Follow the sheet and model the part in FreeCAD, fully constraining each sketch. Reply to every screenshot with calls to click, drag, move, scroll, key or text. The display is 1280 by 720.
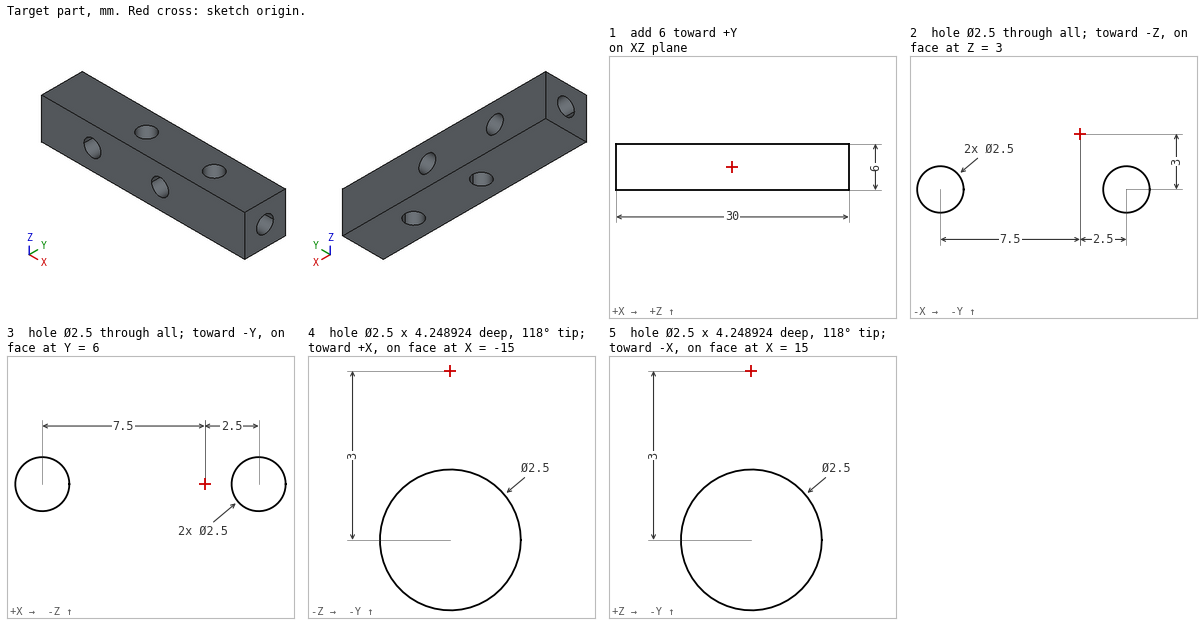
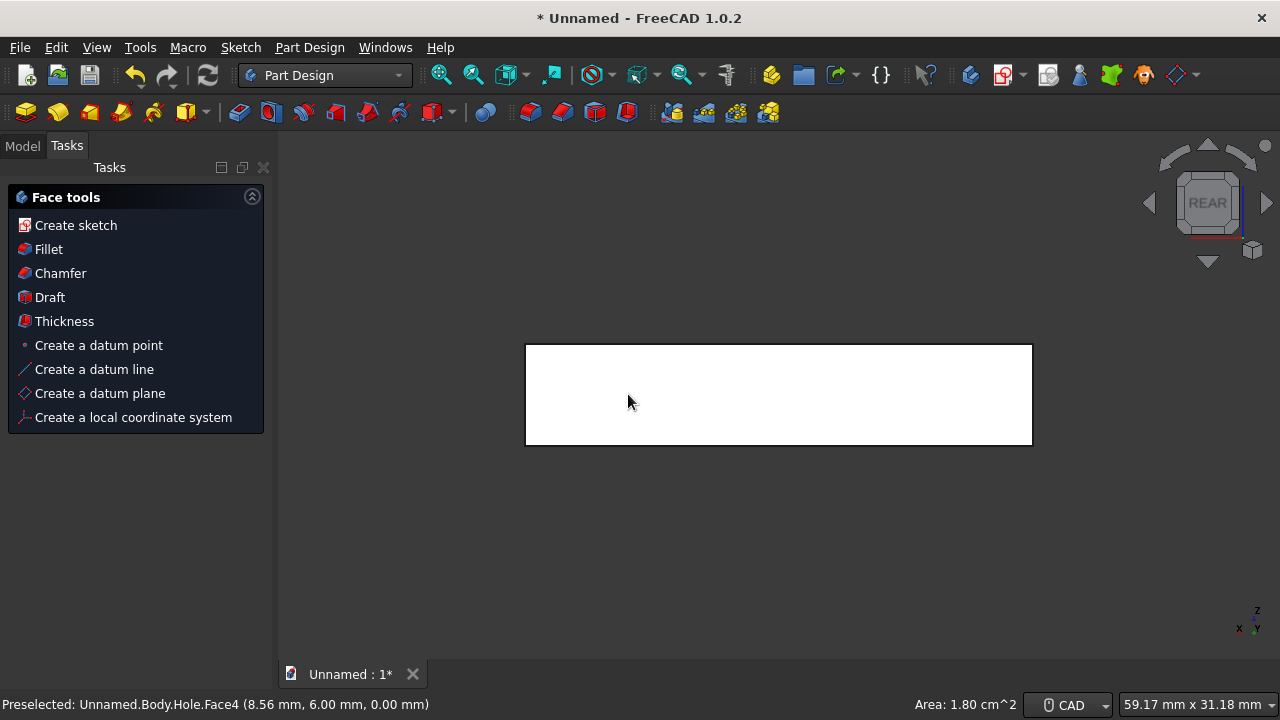
click(1004, 76)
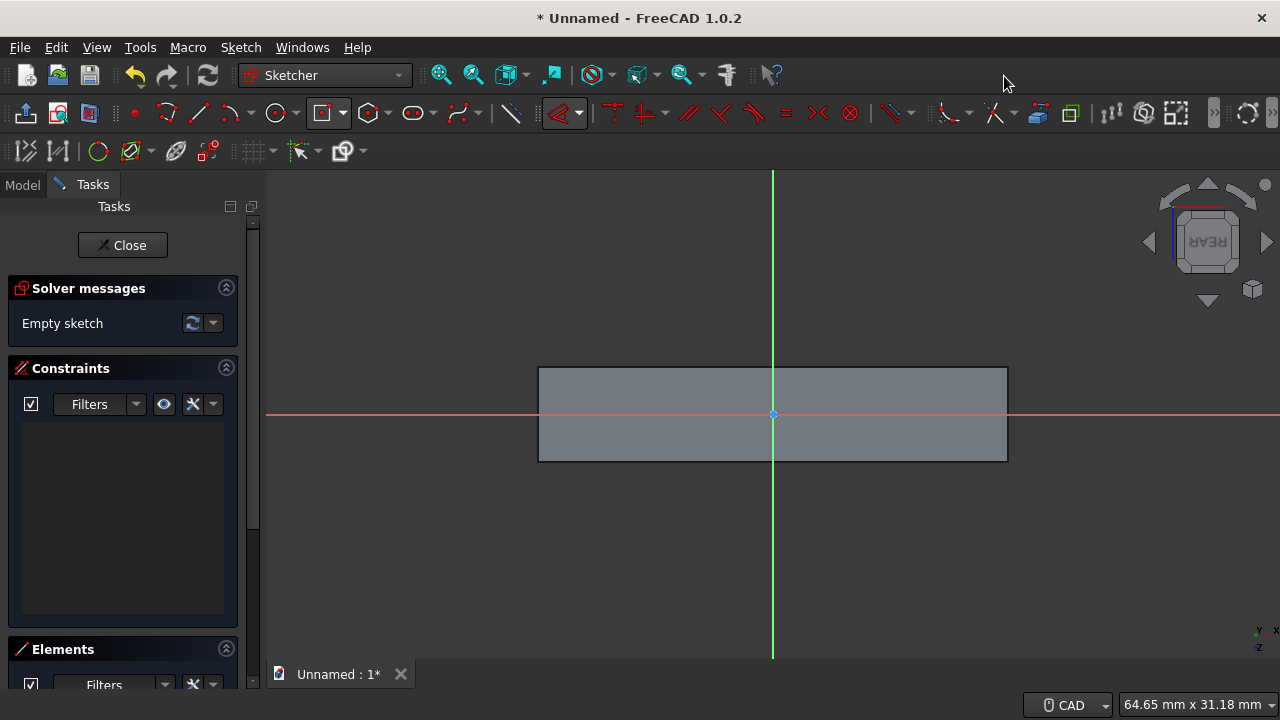
scroll(751, 414, up, 5)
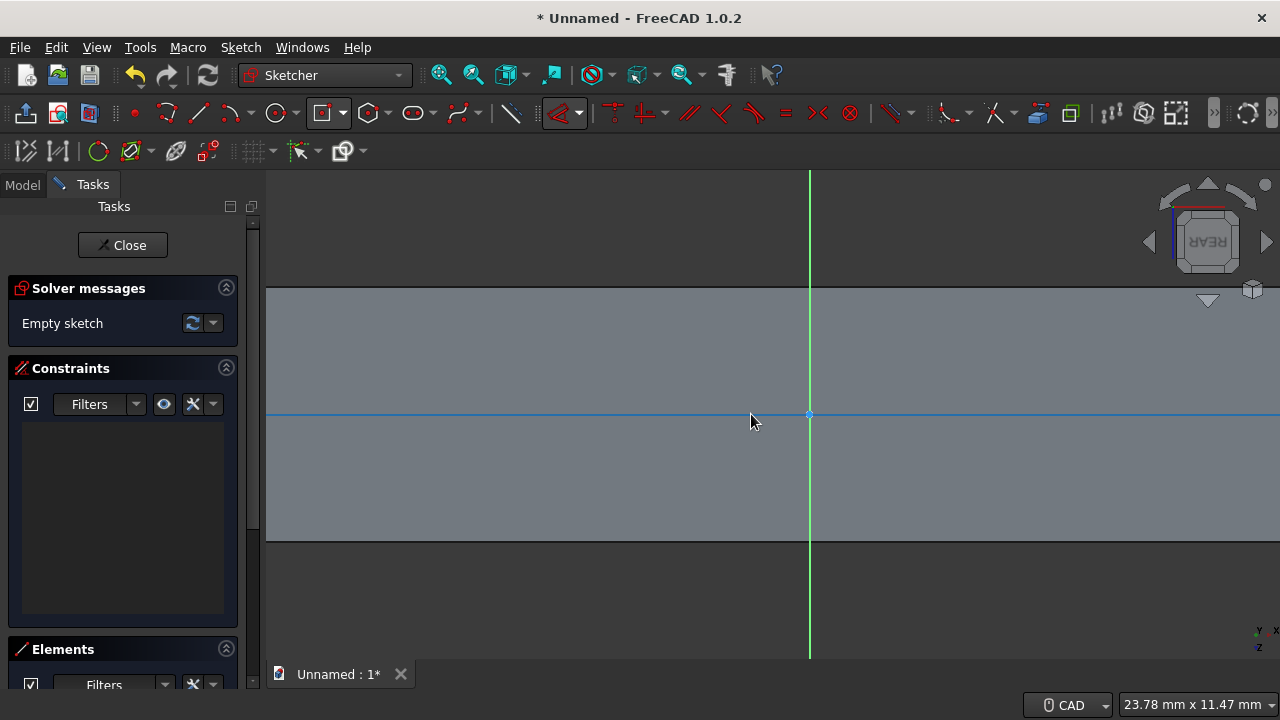
click(276, 114)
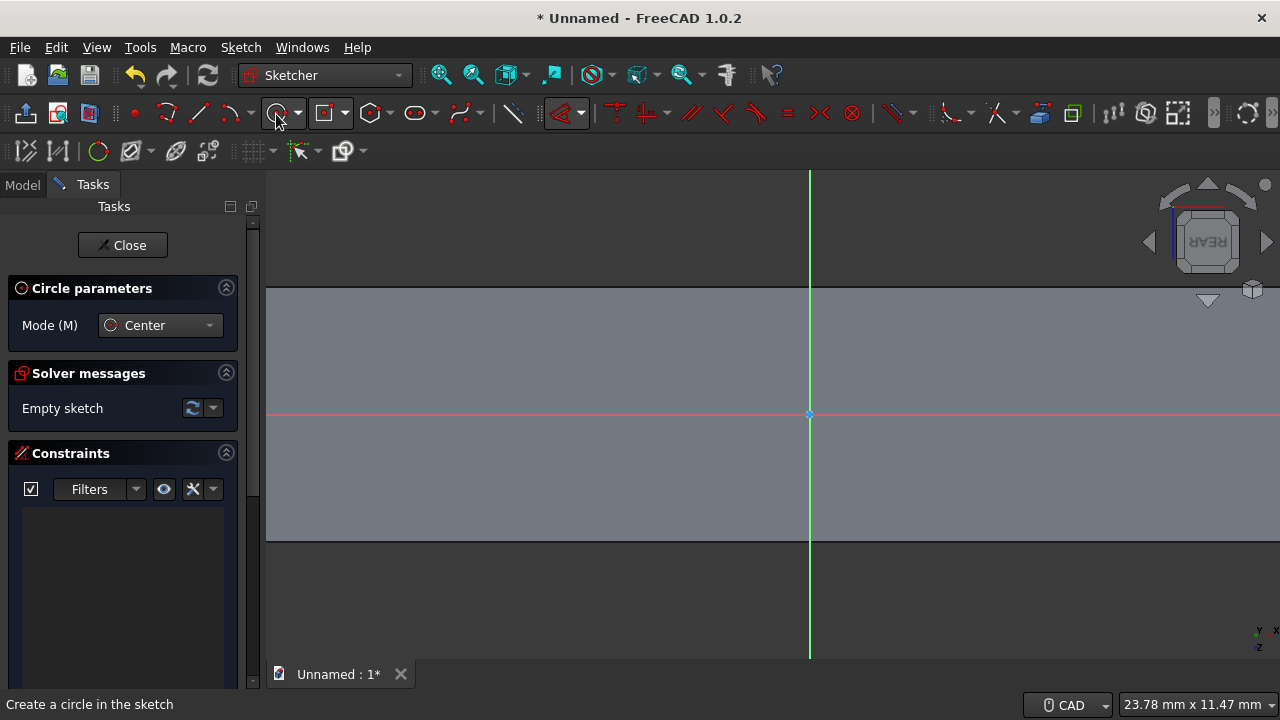
click(917, 414)
move(954, 377)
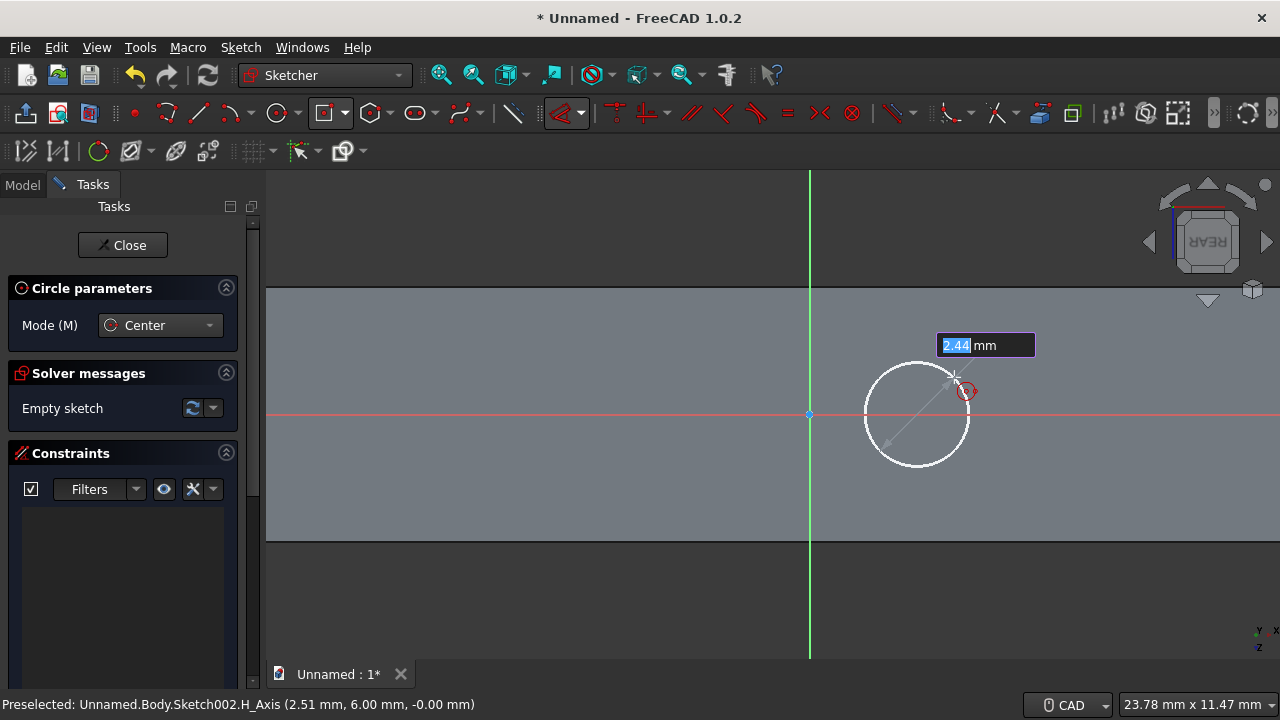
text(2.5)
key(Return)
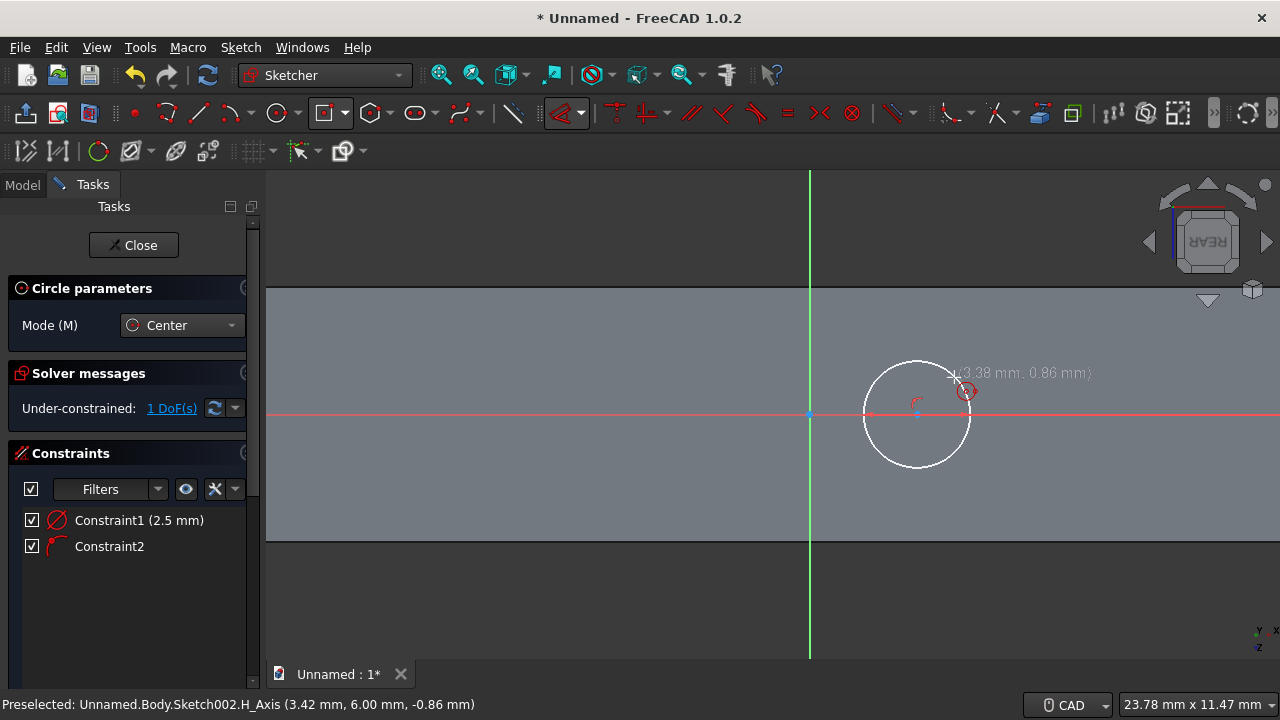
click(490, 414)
move(528, 377)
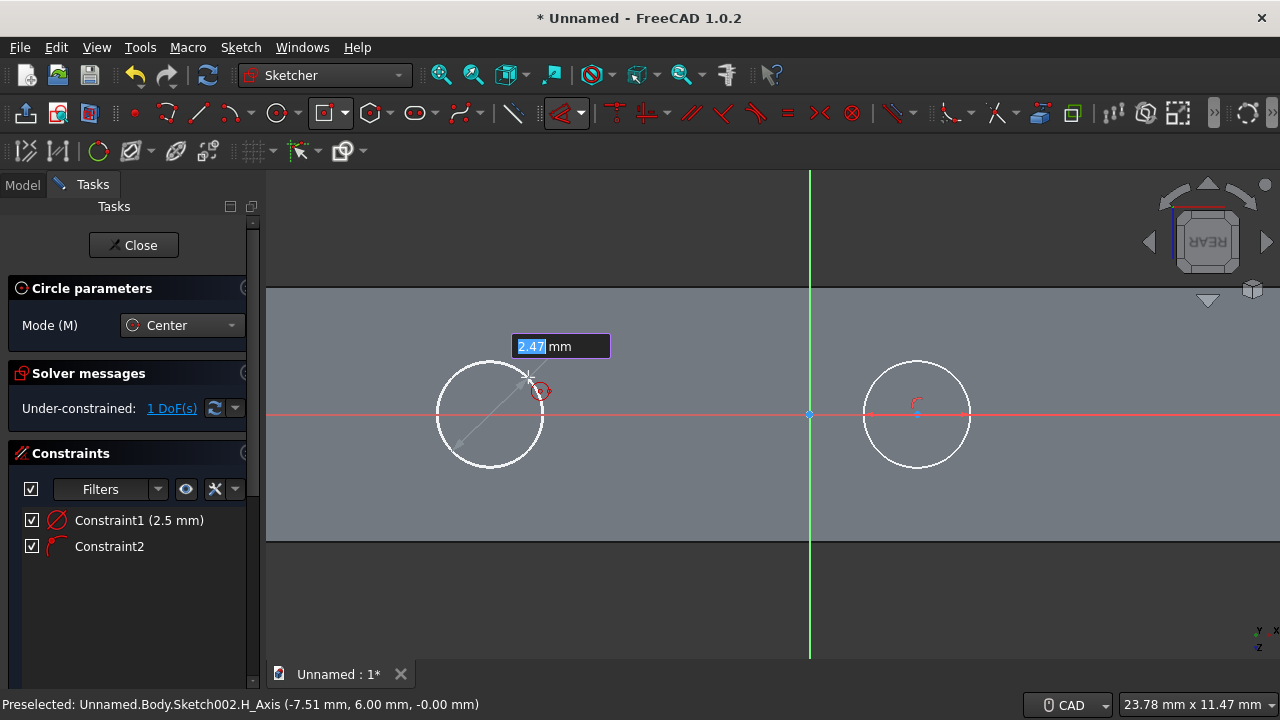
text(2.5)
key(Return)
key(Escape)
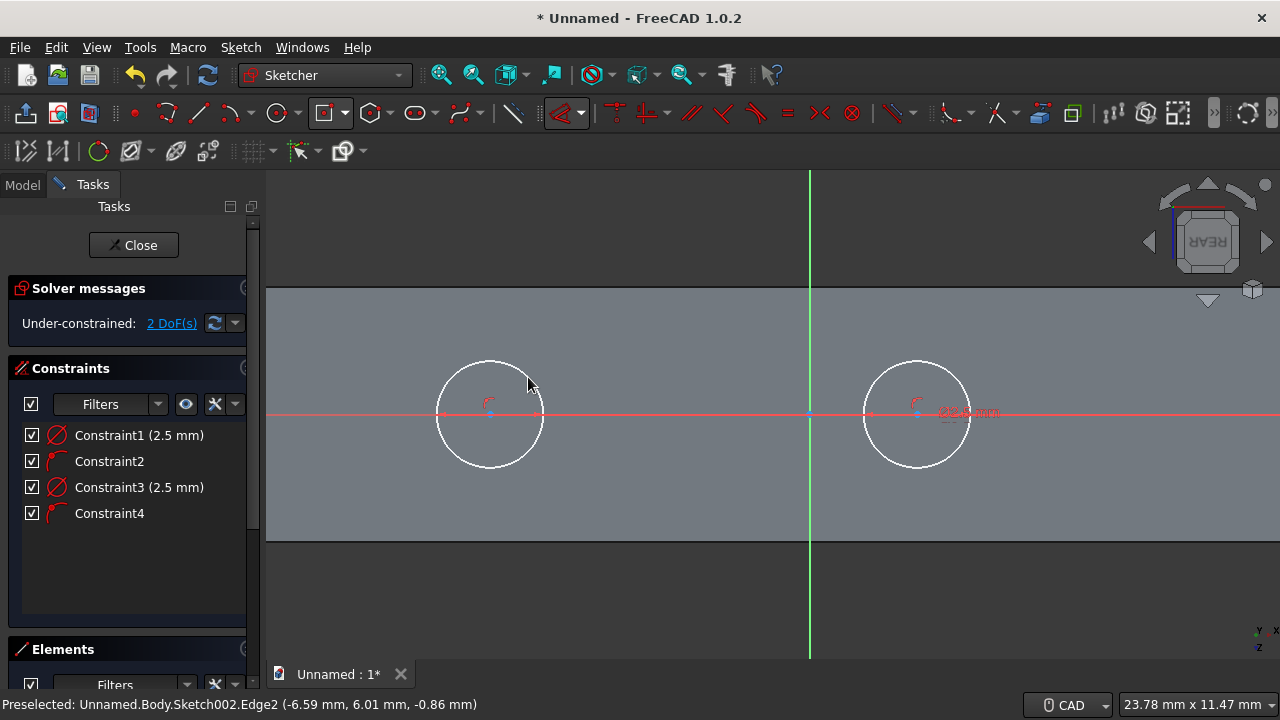
click(917, 414)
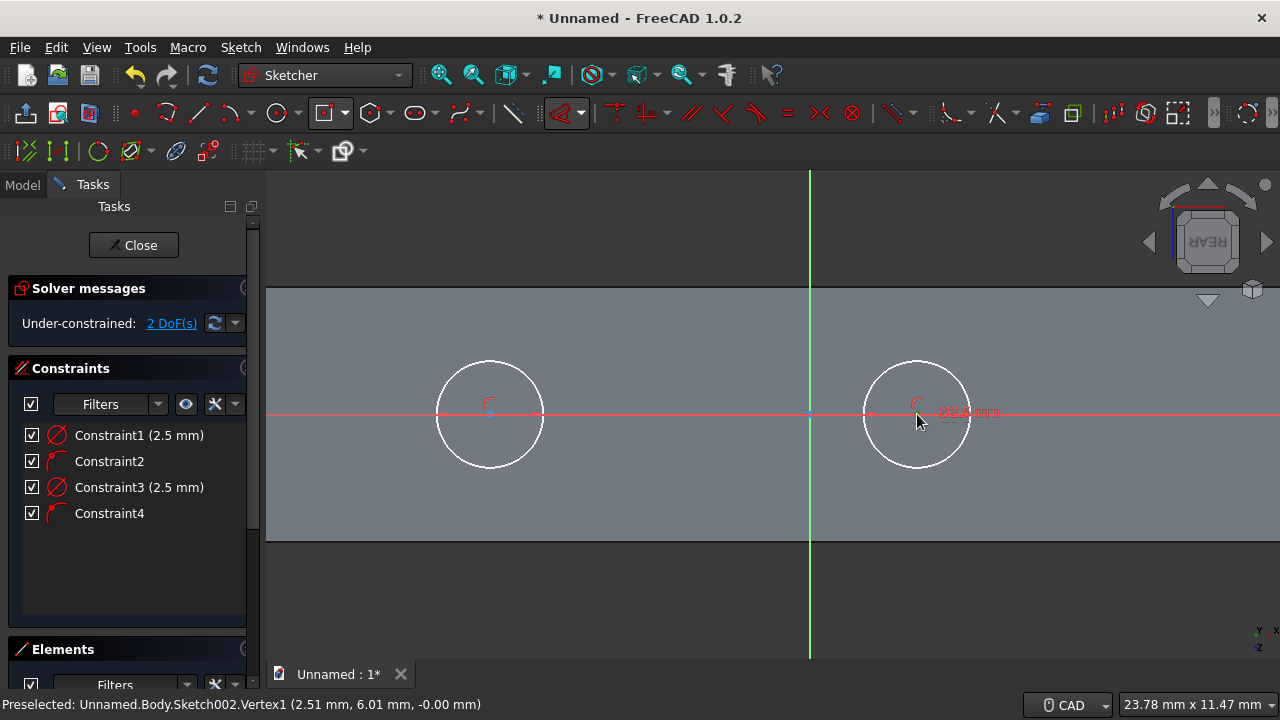
key(l)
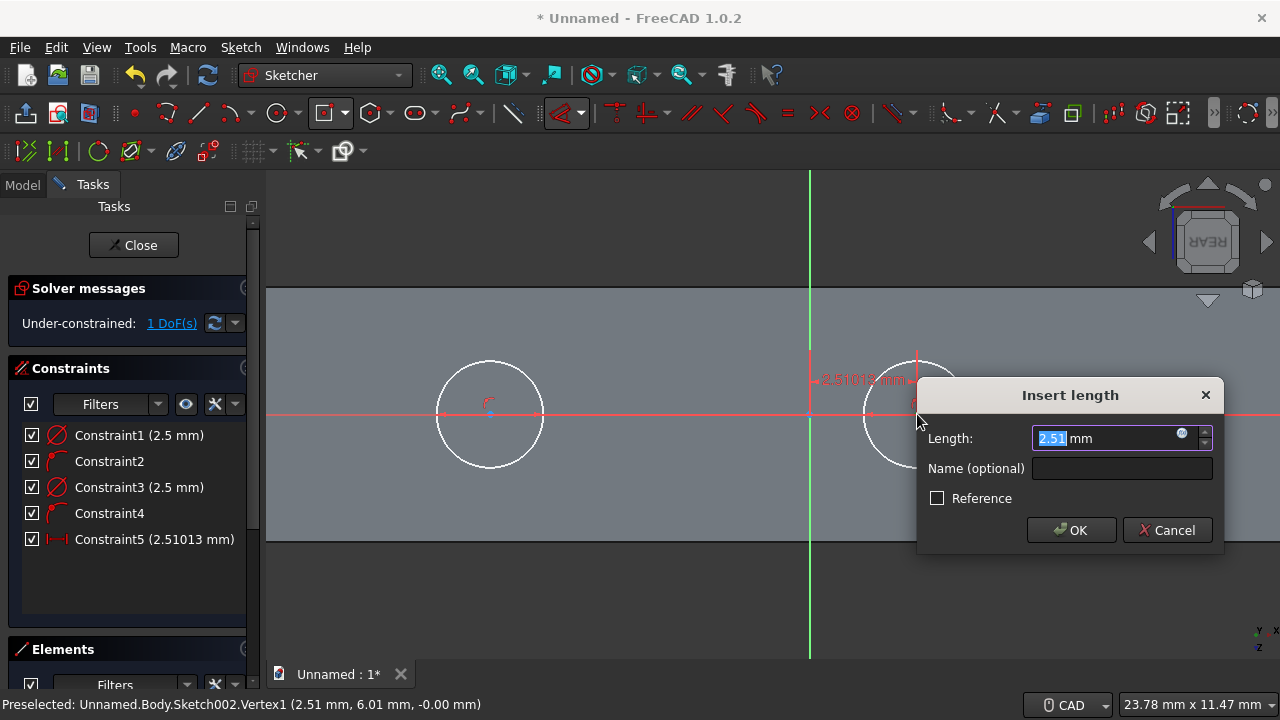
text(2.5)
key(Return)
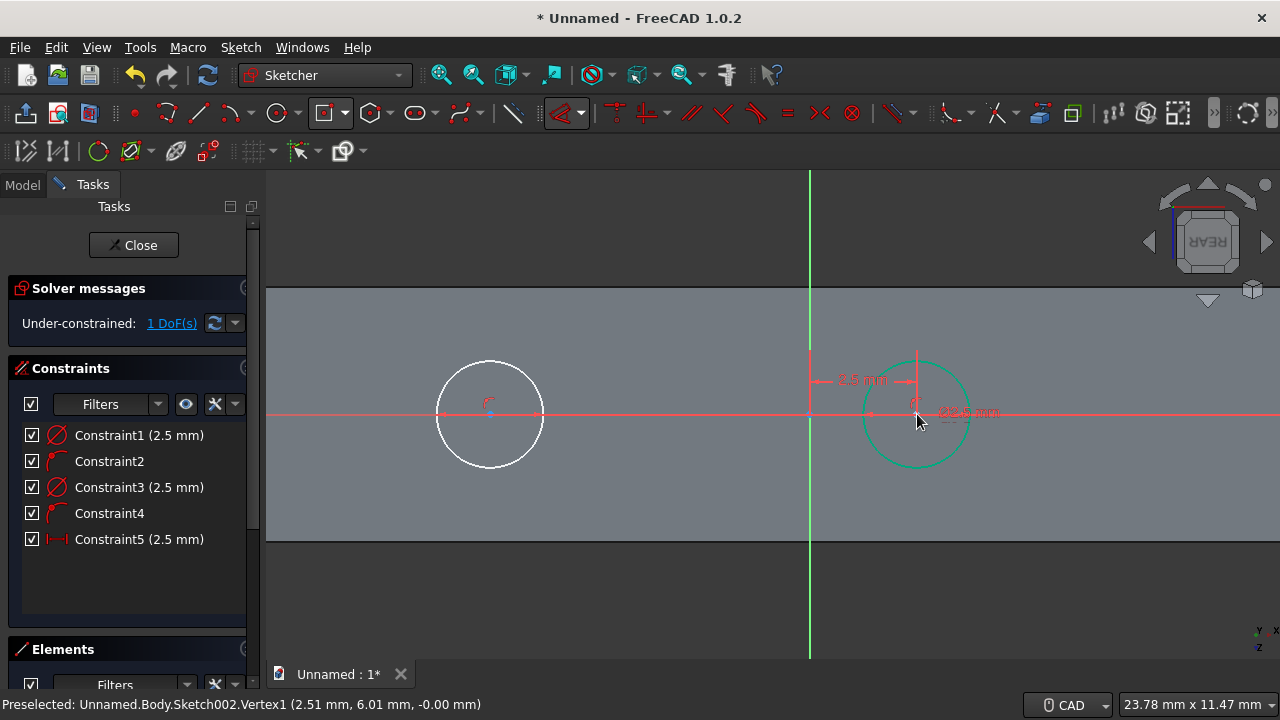
click(490, 414)